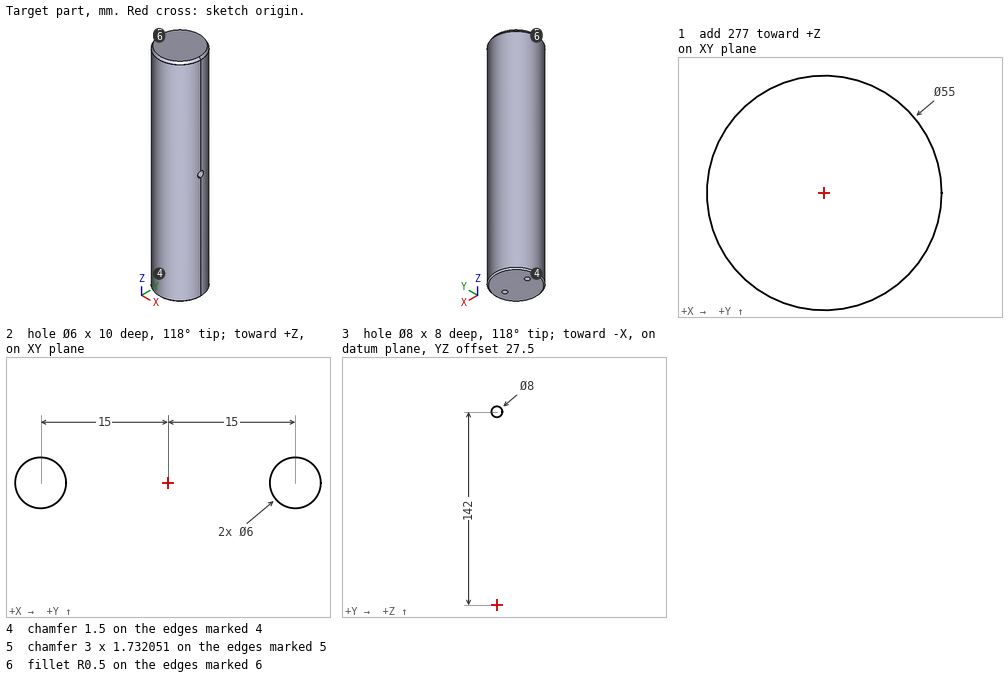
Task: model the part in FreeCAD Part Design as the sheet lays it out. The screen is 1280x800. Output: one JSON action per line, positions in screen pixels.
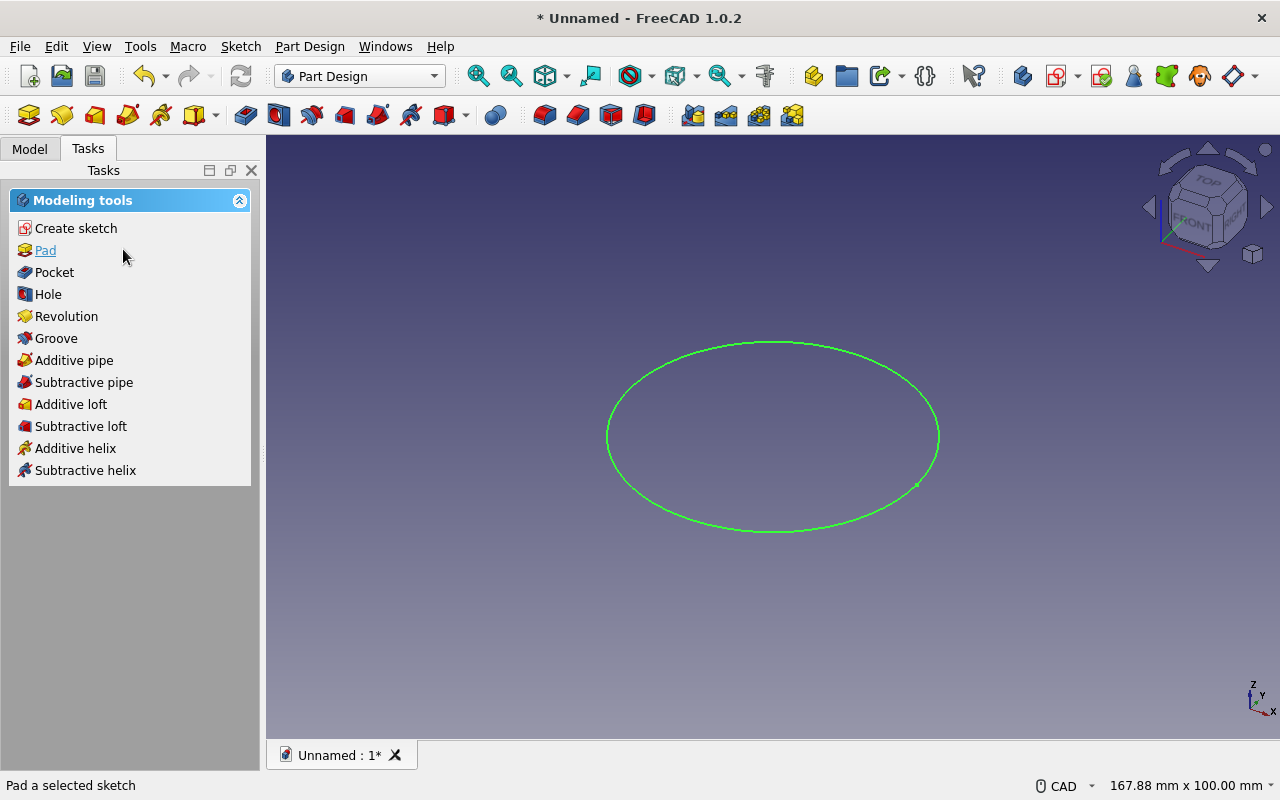
{"action": "left_click", "coordinate": [29, 116]}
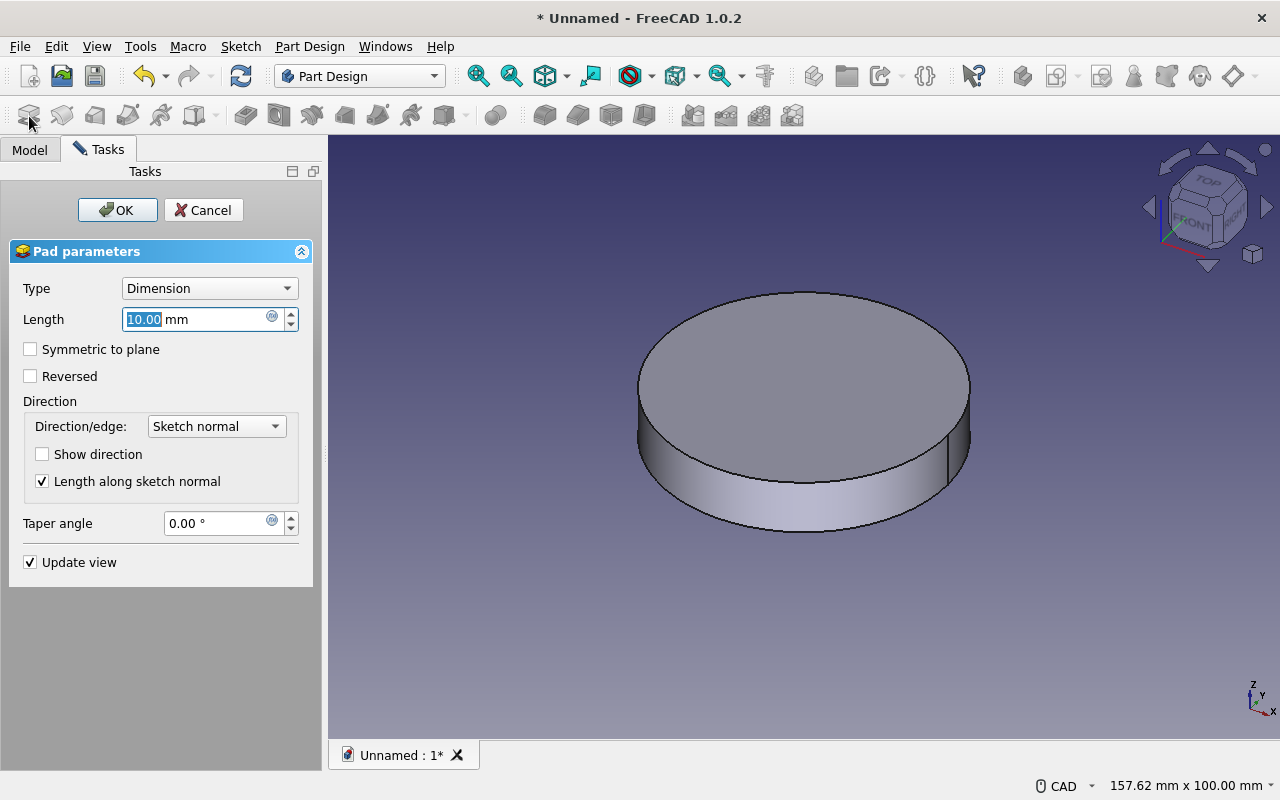
{"action": "type", "text": "277"}
{"action": "key", "text": "Tab"}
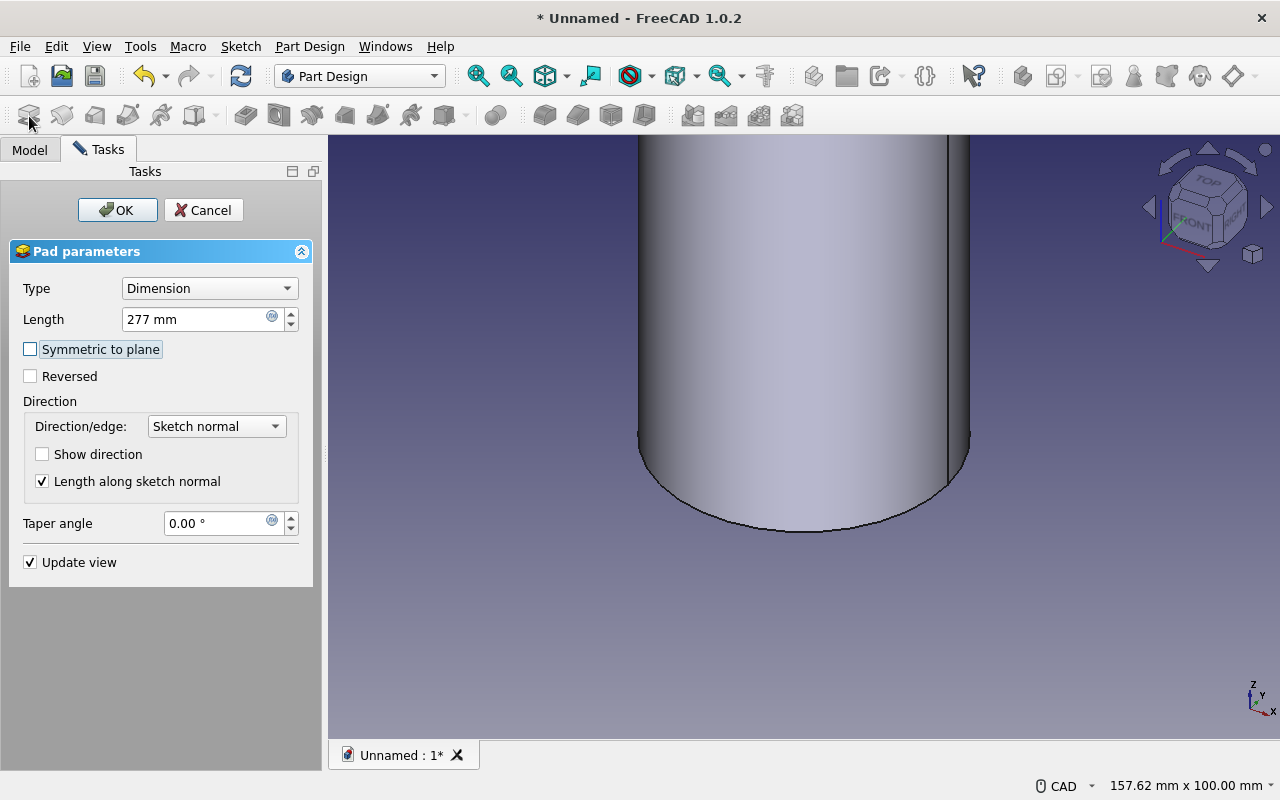
{"action": "left_click", "coordinate": [118, 210]}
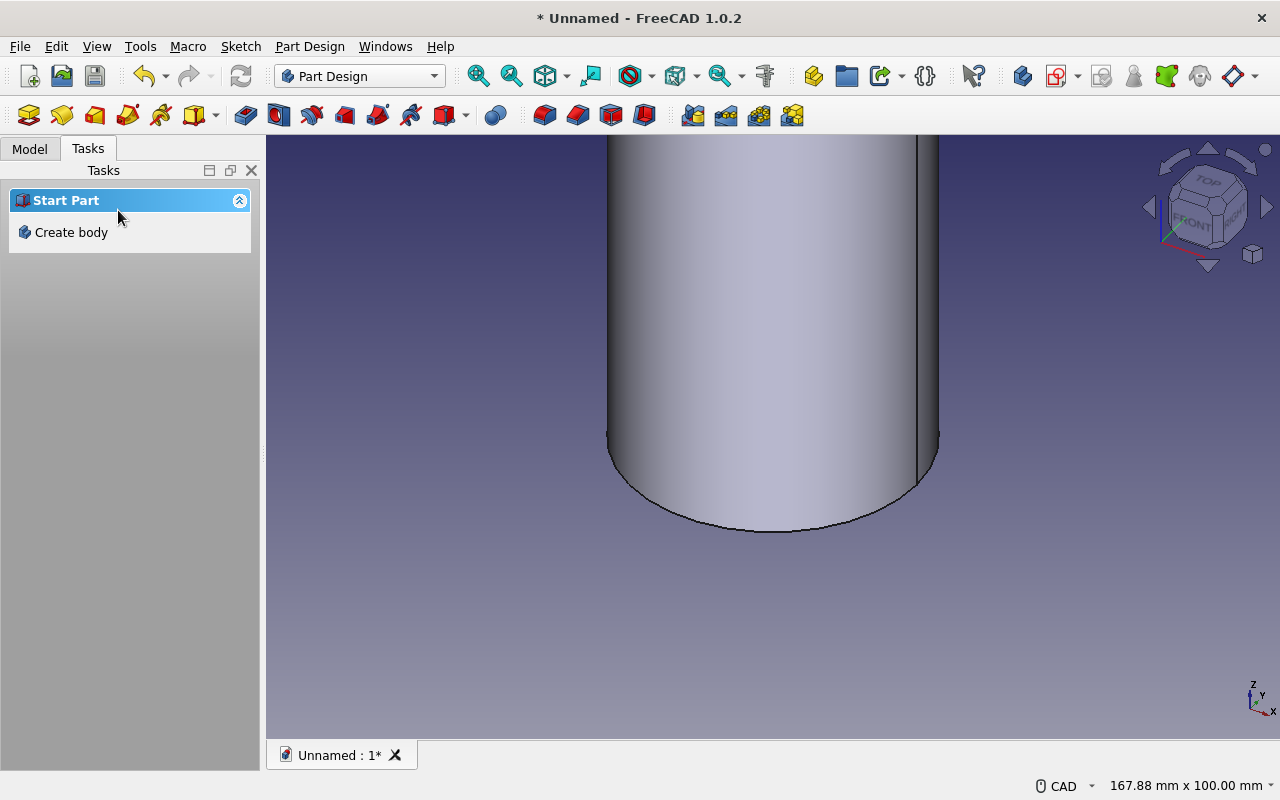
{"action": "left_click", "coordinate": [479, 76]}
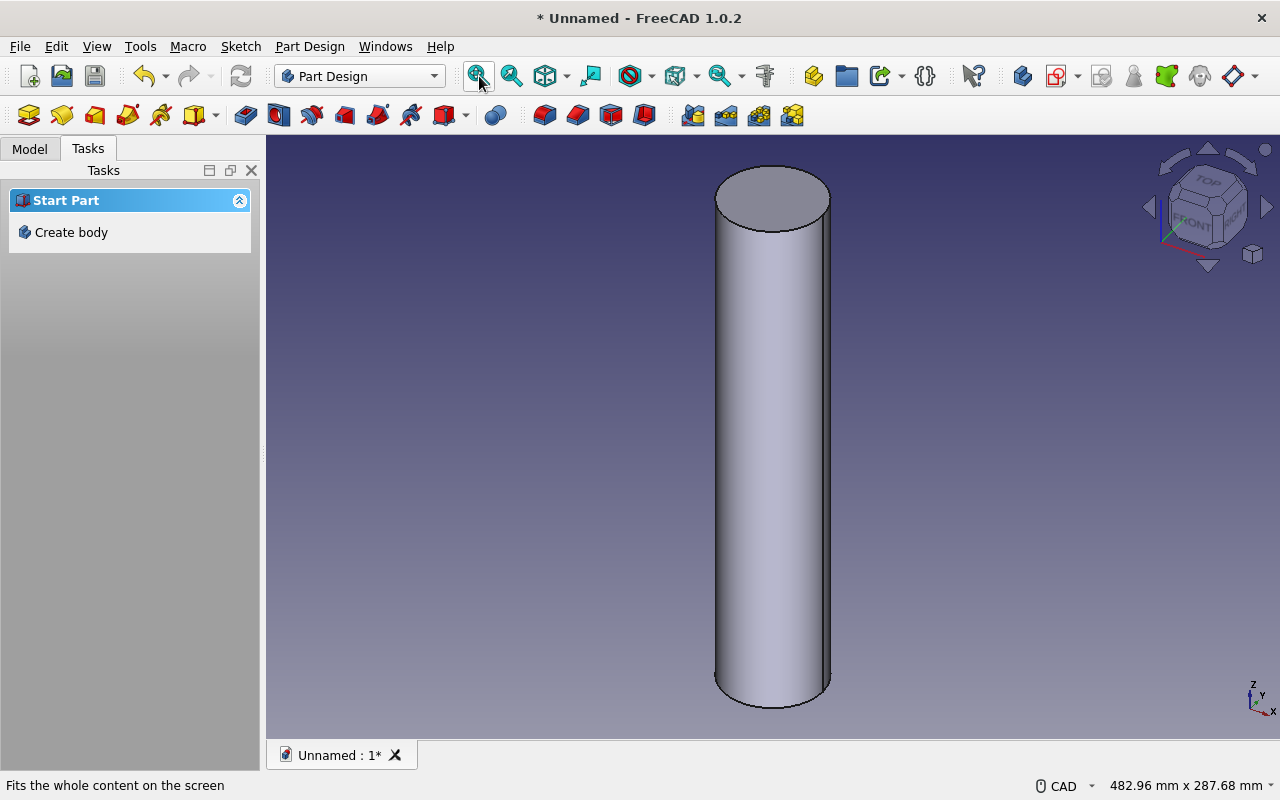
{"action": "left_click", "coordinate": [1056, 76]}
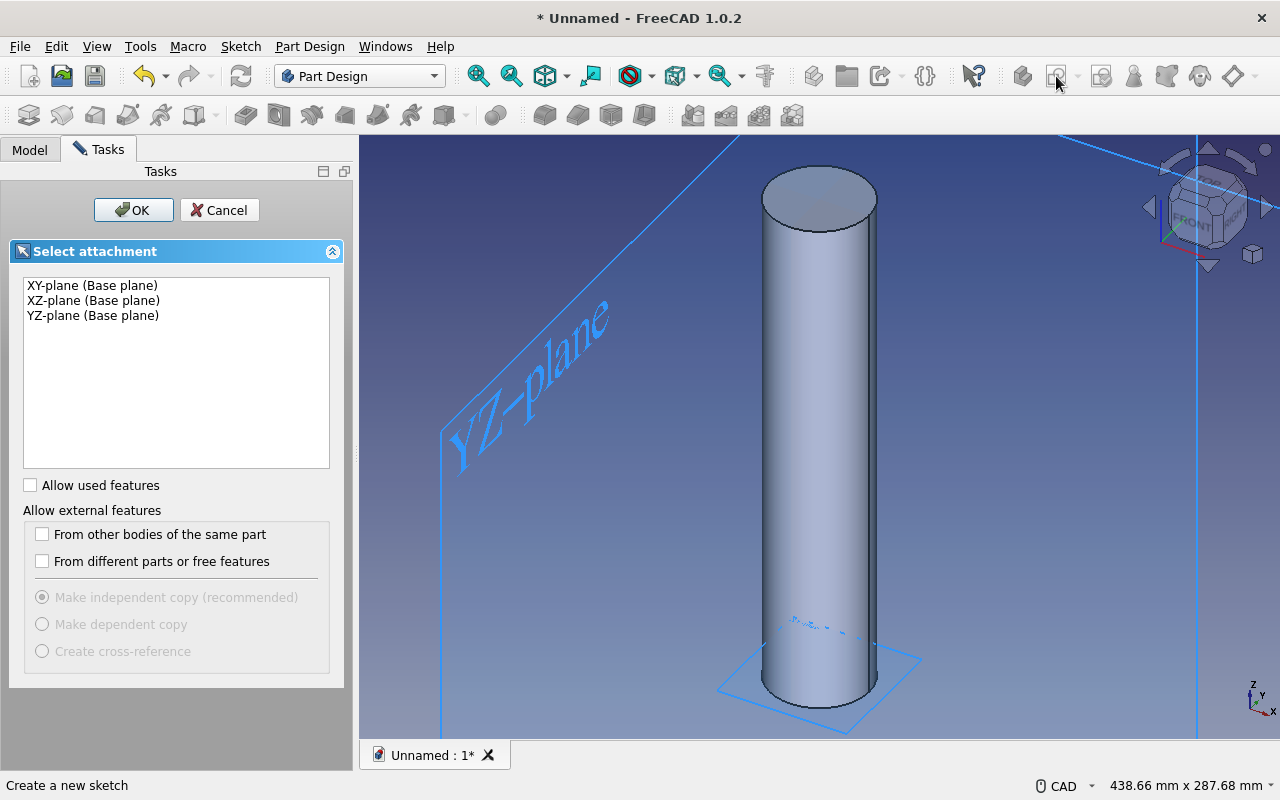
{"action": "left_click", "coordinate": [84, 286]}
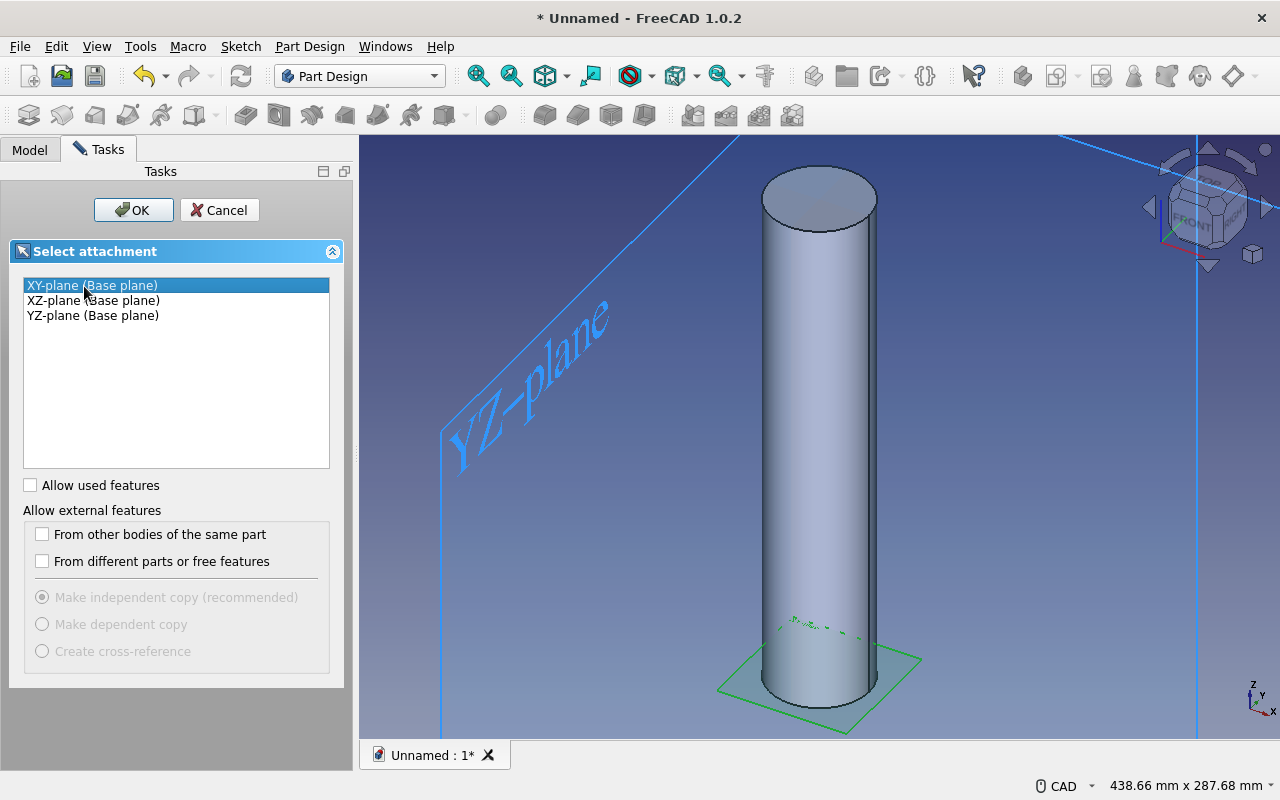
{"action": "left_click", "coordinate": [134, 210]}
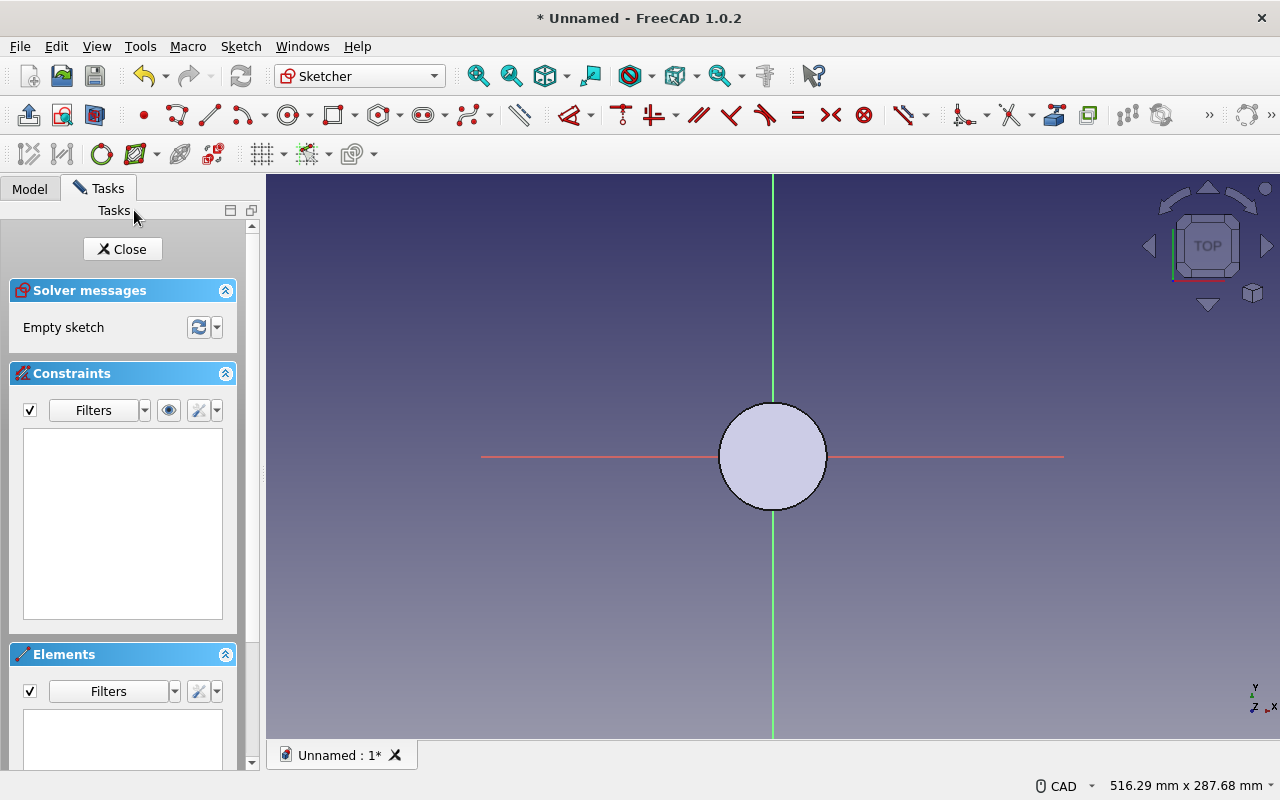
{"action": "key", "text": "q s"}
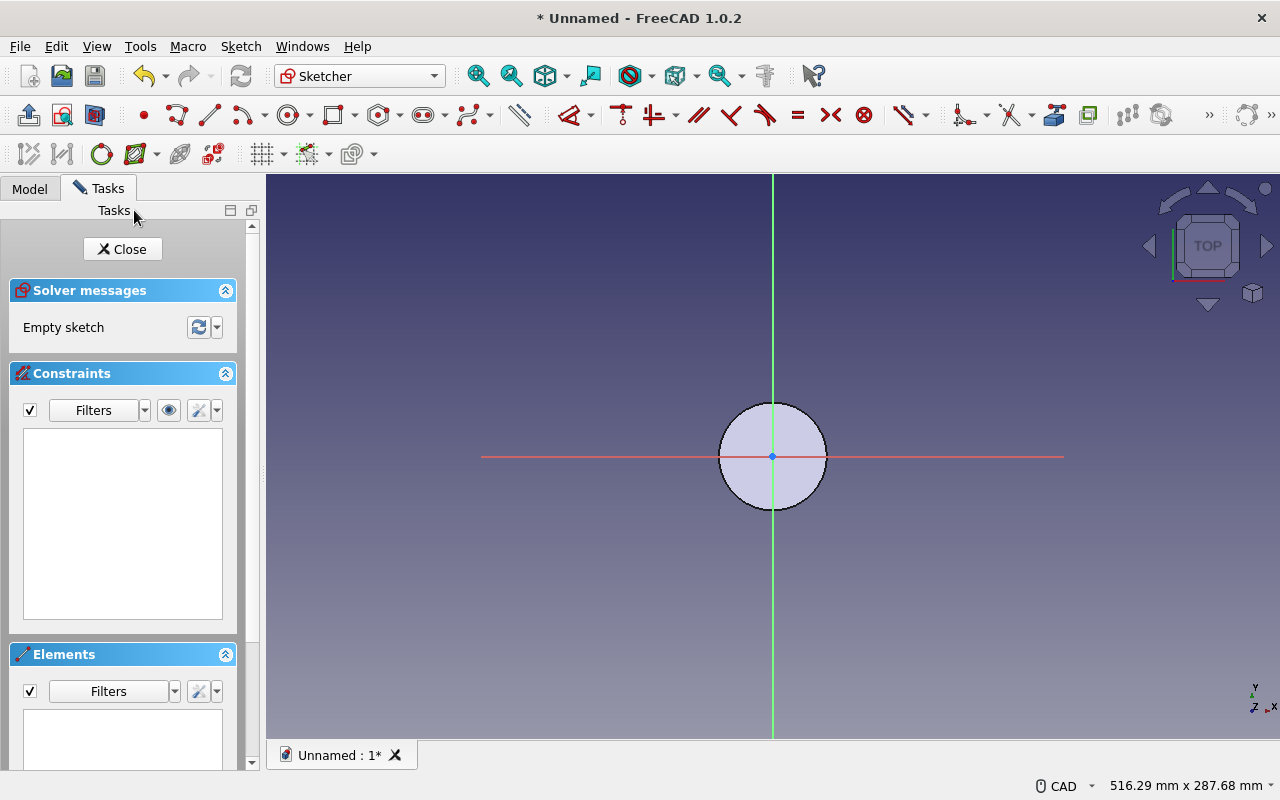
{"action": "scroll", "coordinate": [781, 456], "scroll_direction": "up", "scroll_amount": 11}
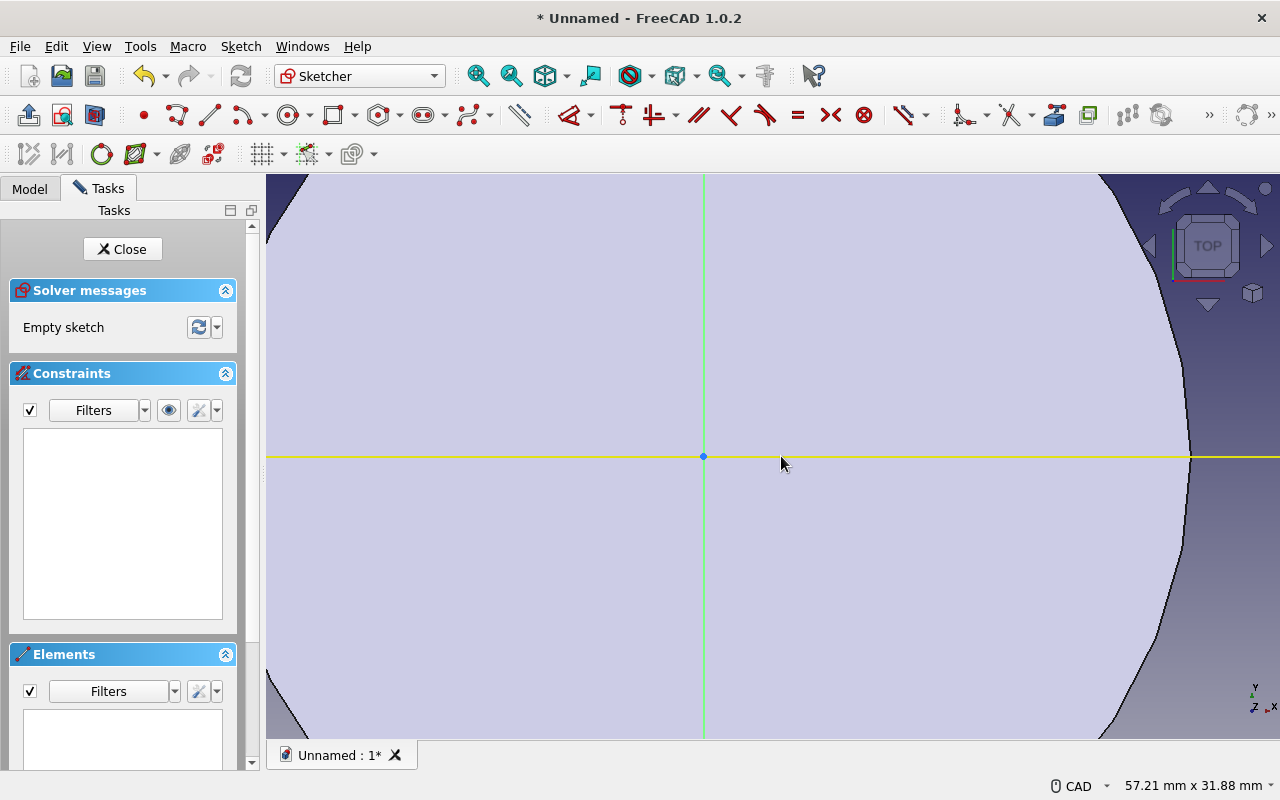
{"action": "key", "text": "g c"}